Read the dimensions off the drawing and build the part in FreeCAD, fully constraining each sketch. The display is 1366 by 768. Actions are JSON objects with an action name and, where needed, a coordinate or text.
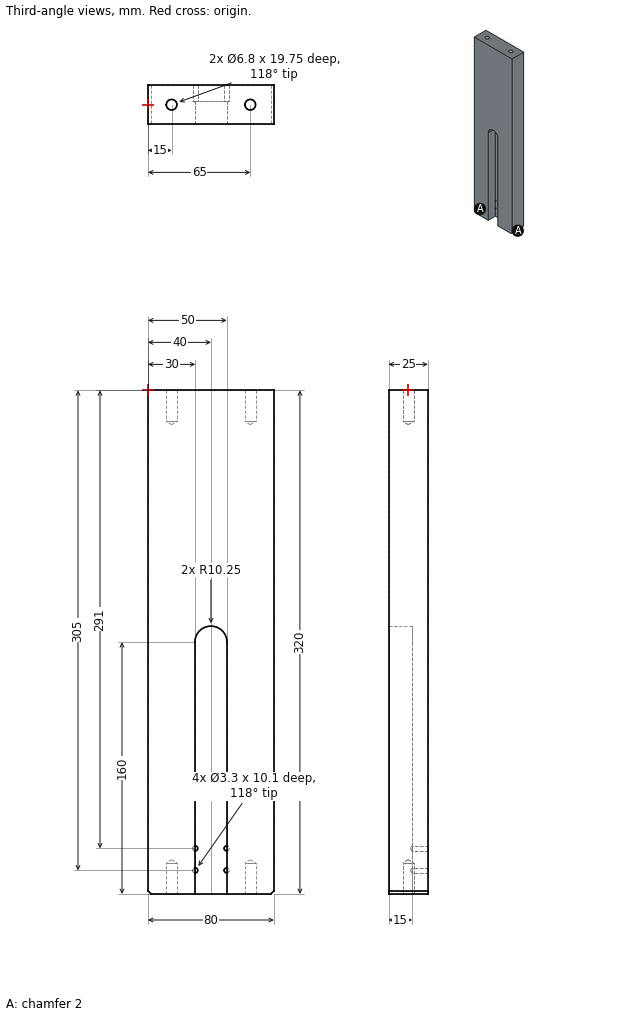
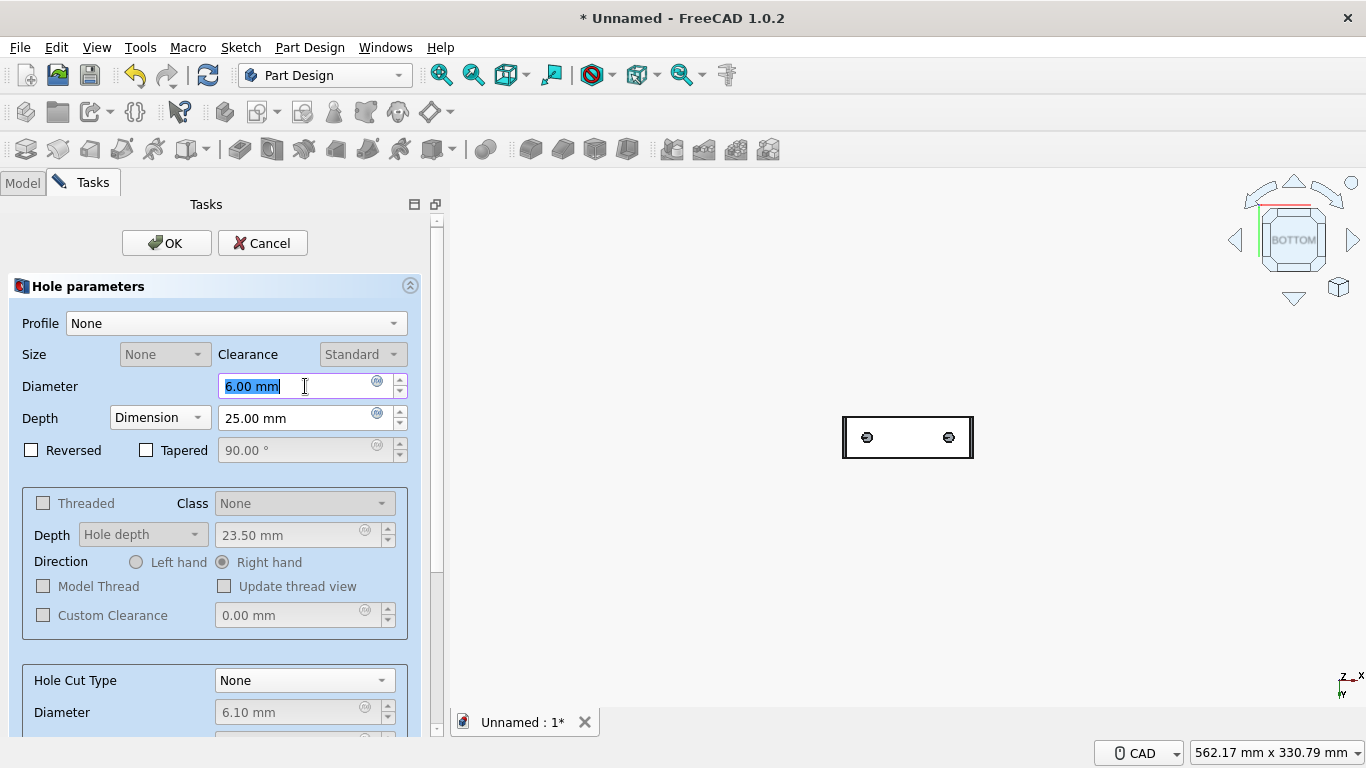
{"action": "type", "text": "6.8"}
{"action": "key", "text": "Tab"}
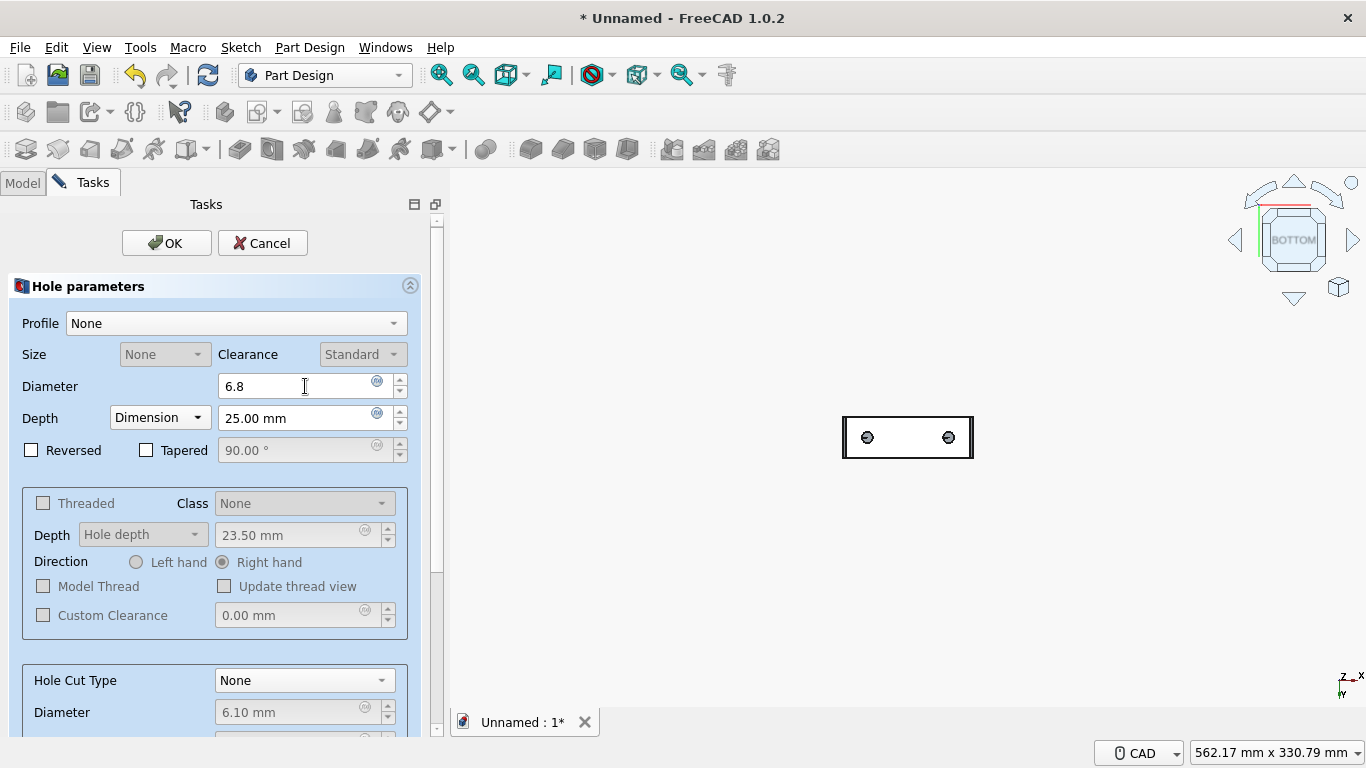
{"action": "triple_click", "coordinate": [305, 418]}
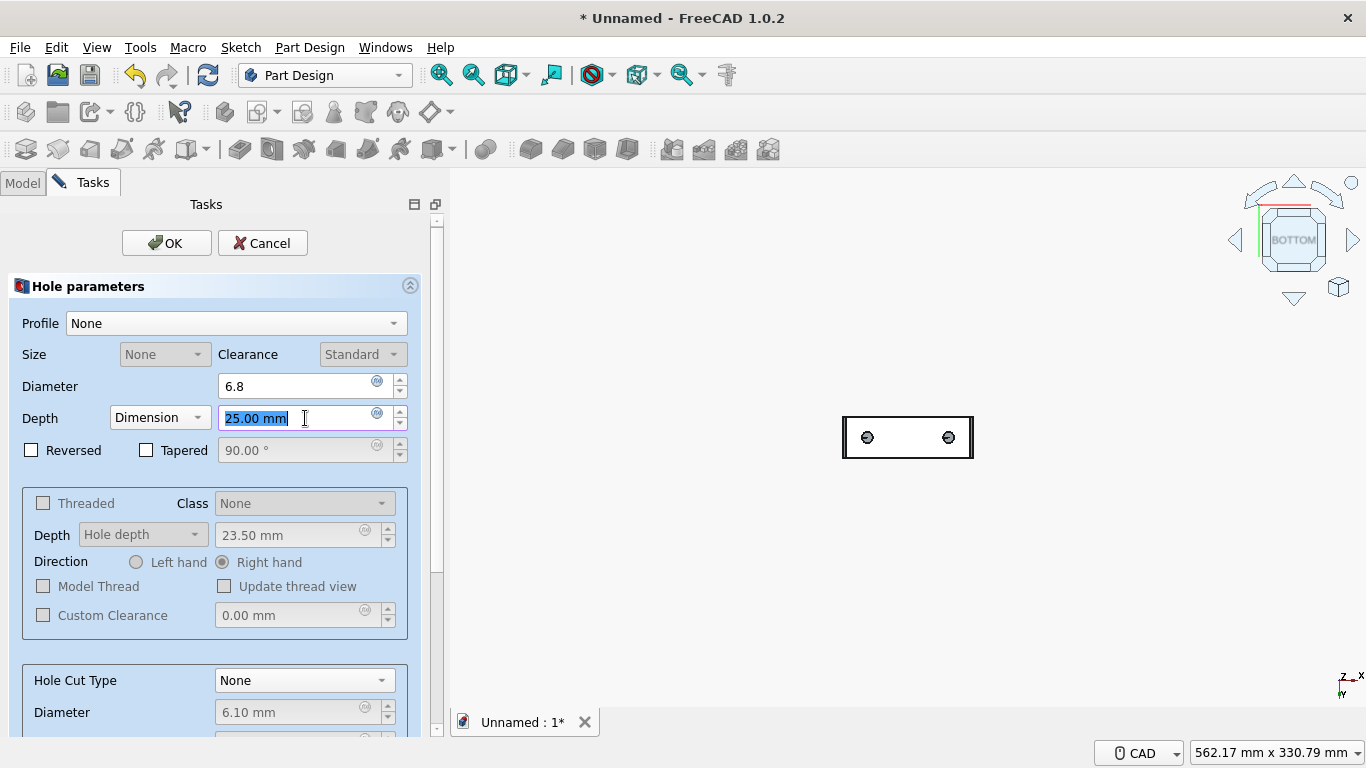
{"action": "type", "text": "19.75"}
{"action": "key", "text": "Tab"}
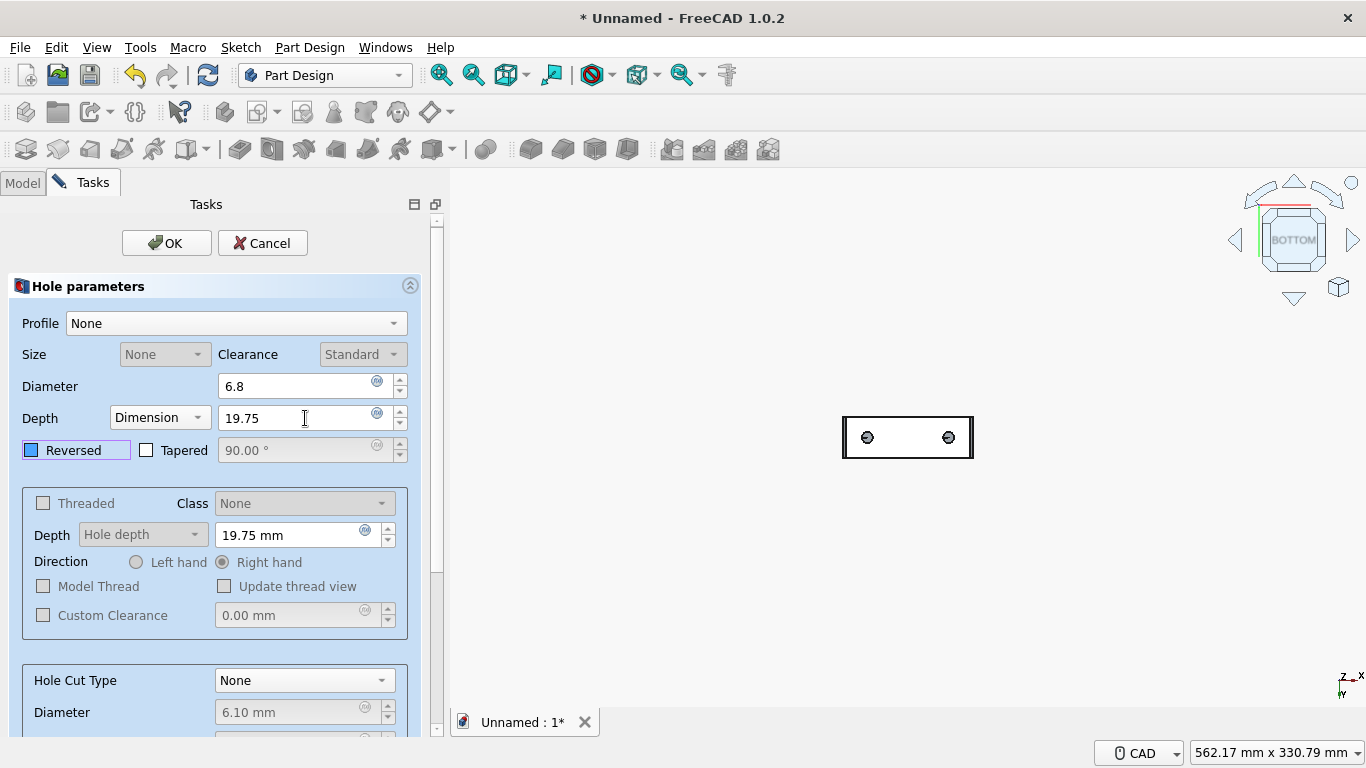
{"action": "left_click", "coordinate": [167, 243]}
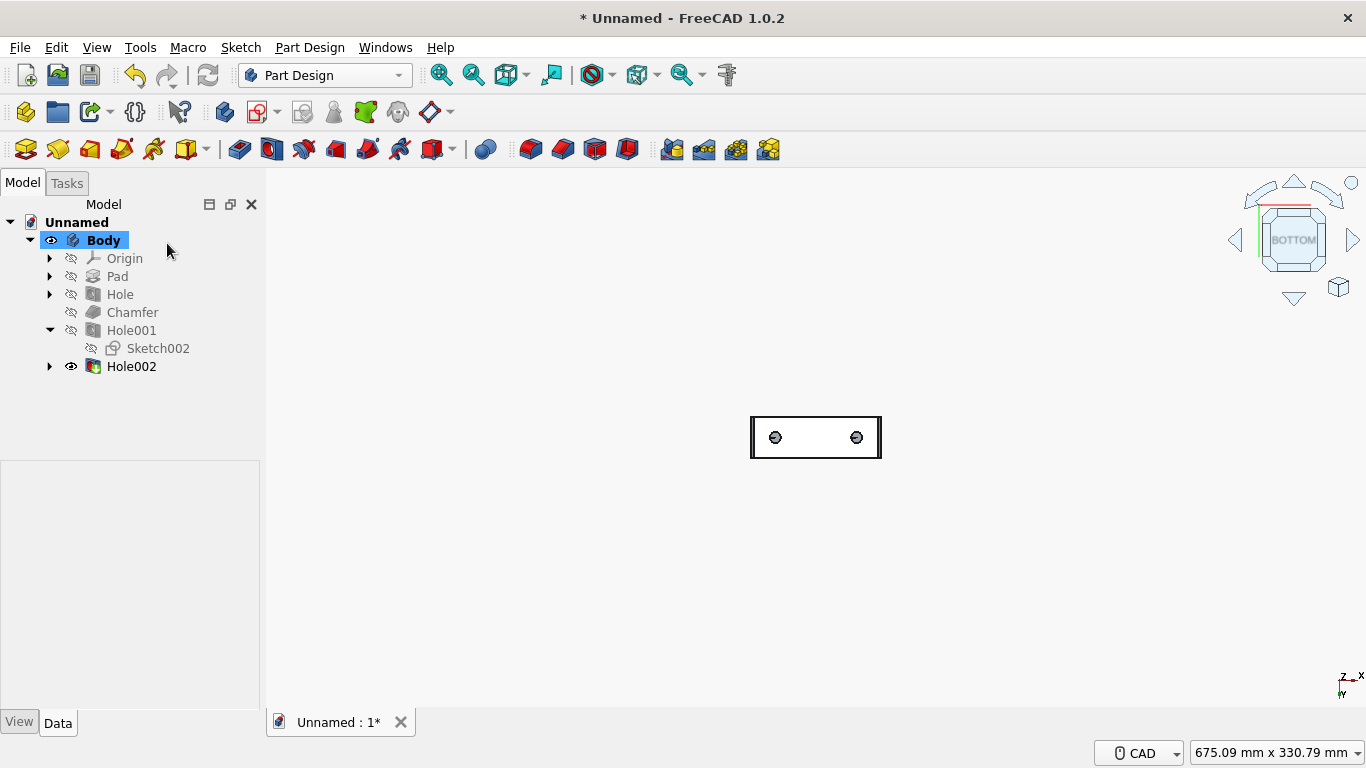
{"action": "left_click", "coordinate": [442, 76]}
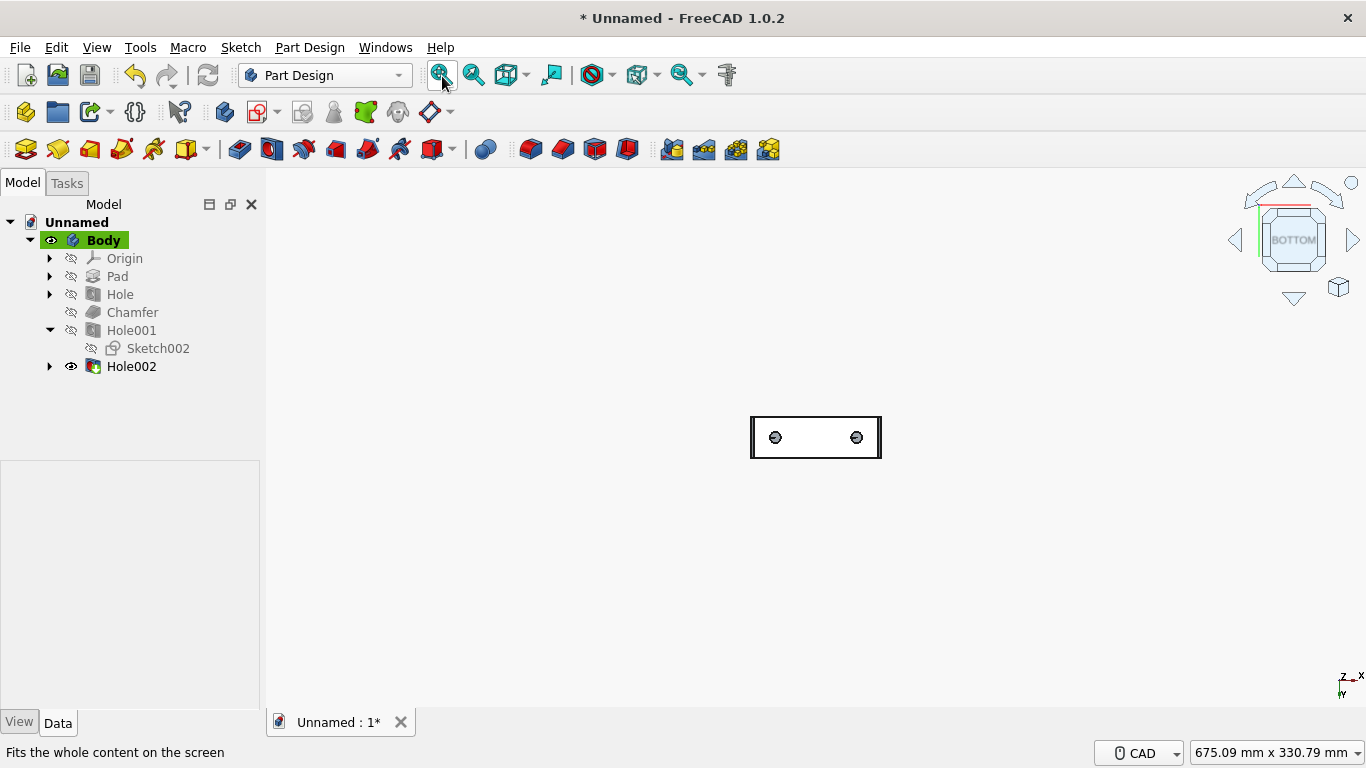
{"action": "key", "text": "0"}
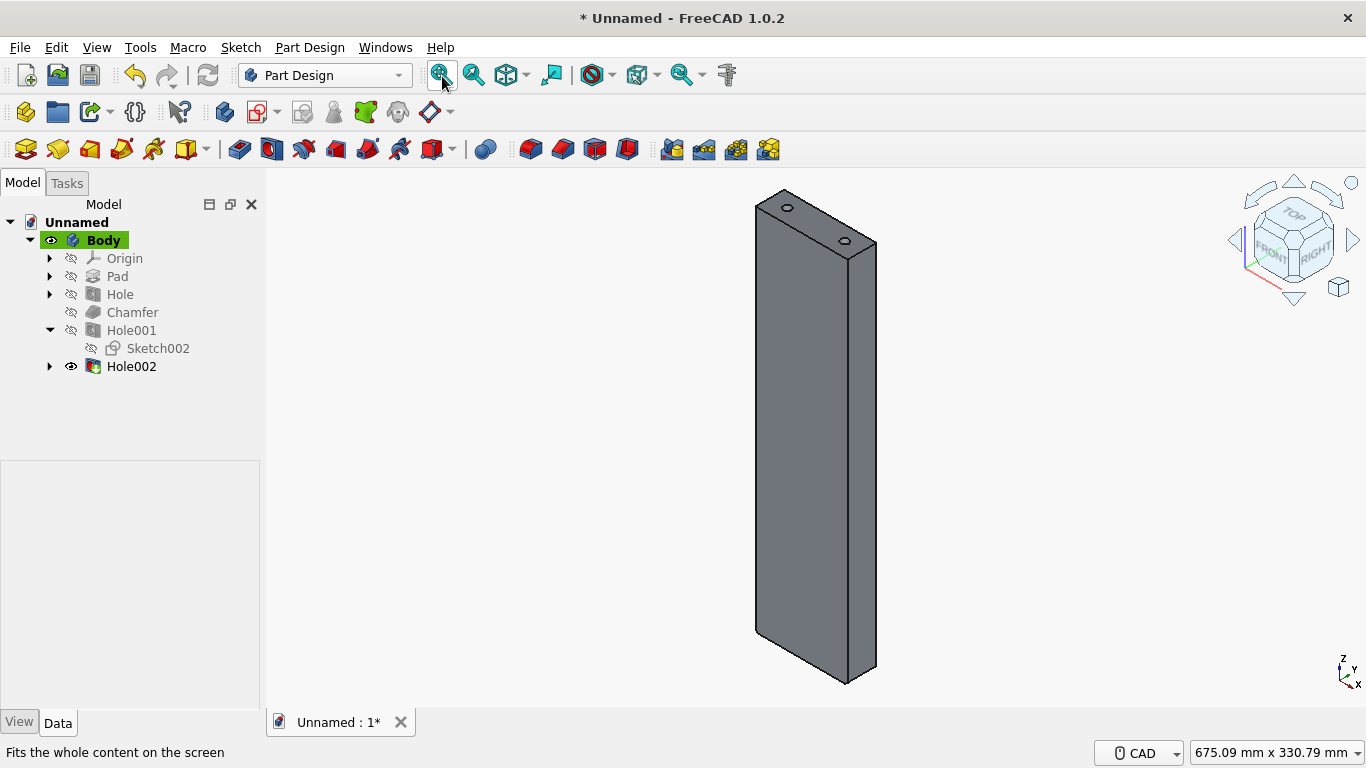
{"action": "left_click", "coordinate": [802, 323]}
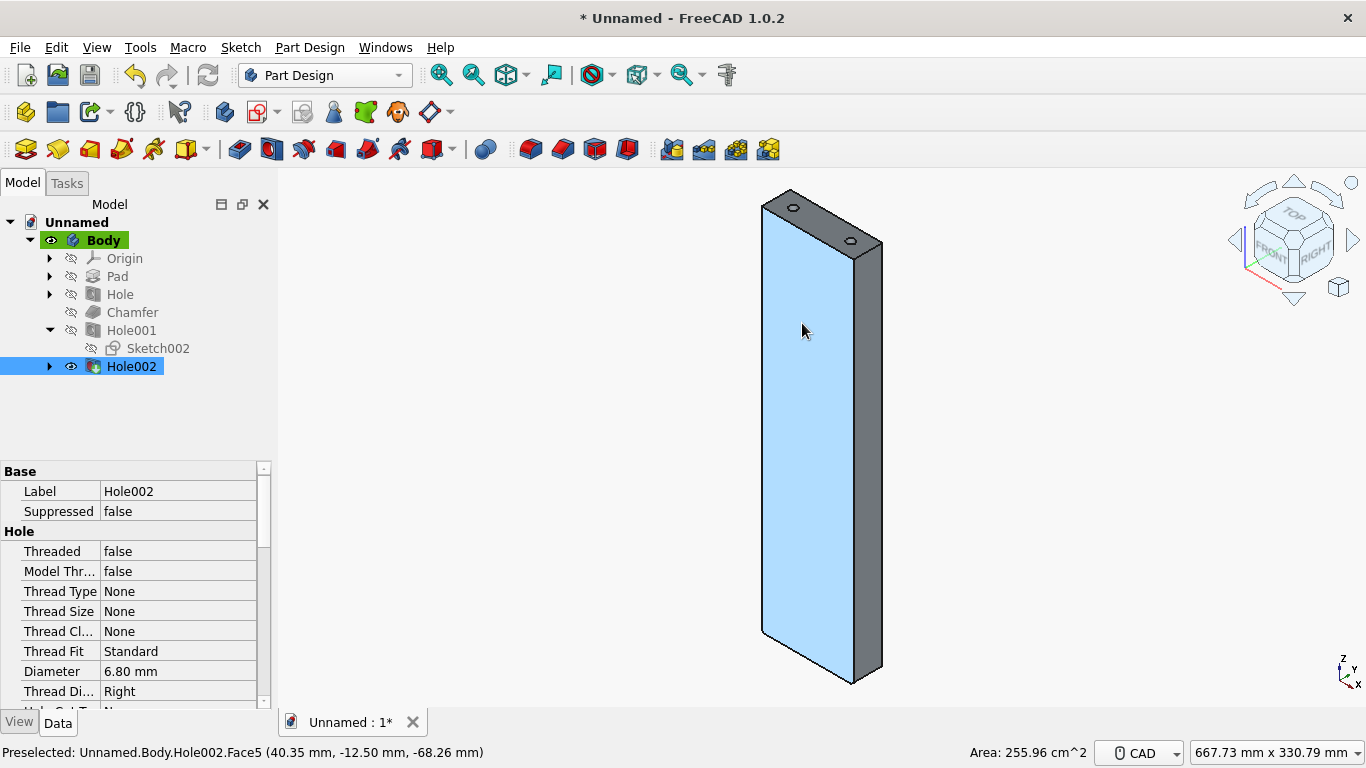
{"action": "left_click", "coordinate": [258, 112]}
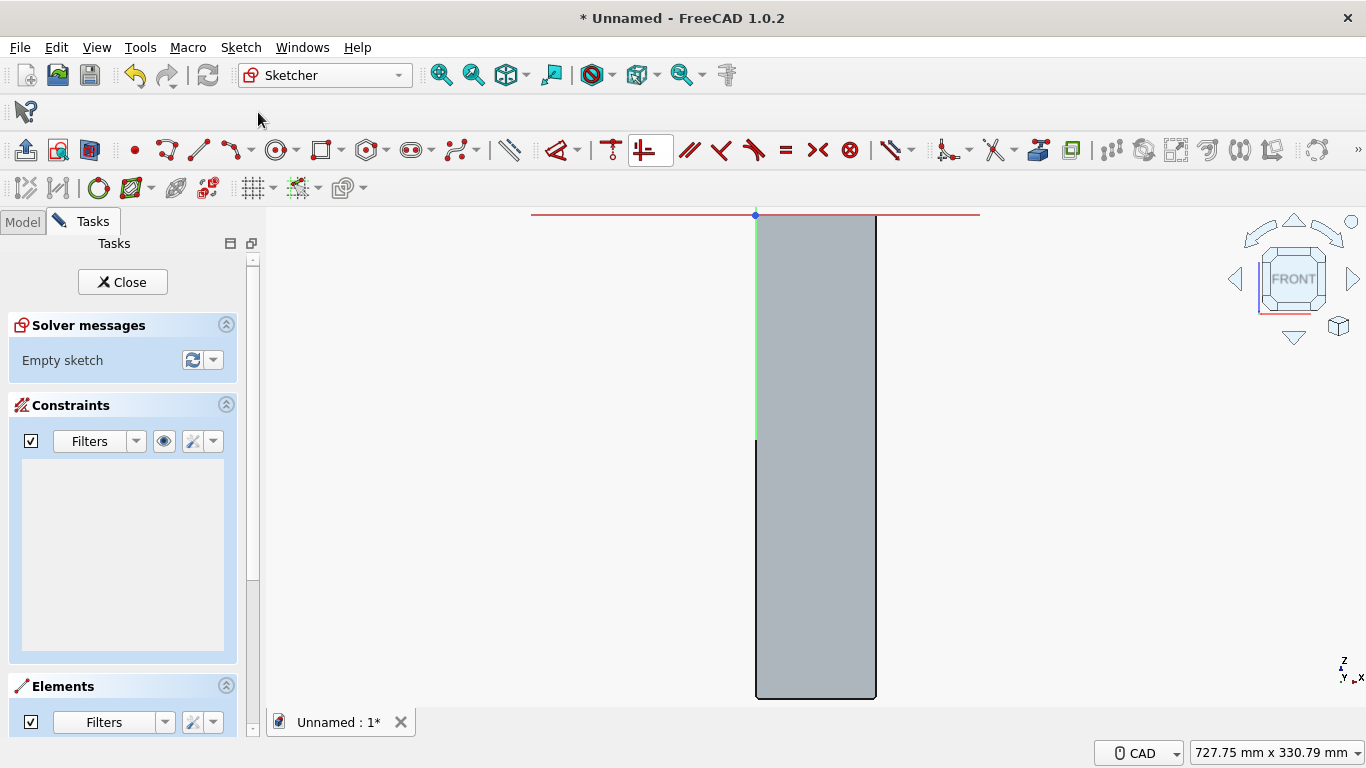
{"action": "scroll", "coordinate": [654, 441], "scroll_direction": "down", "scroll_amount": 2}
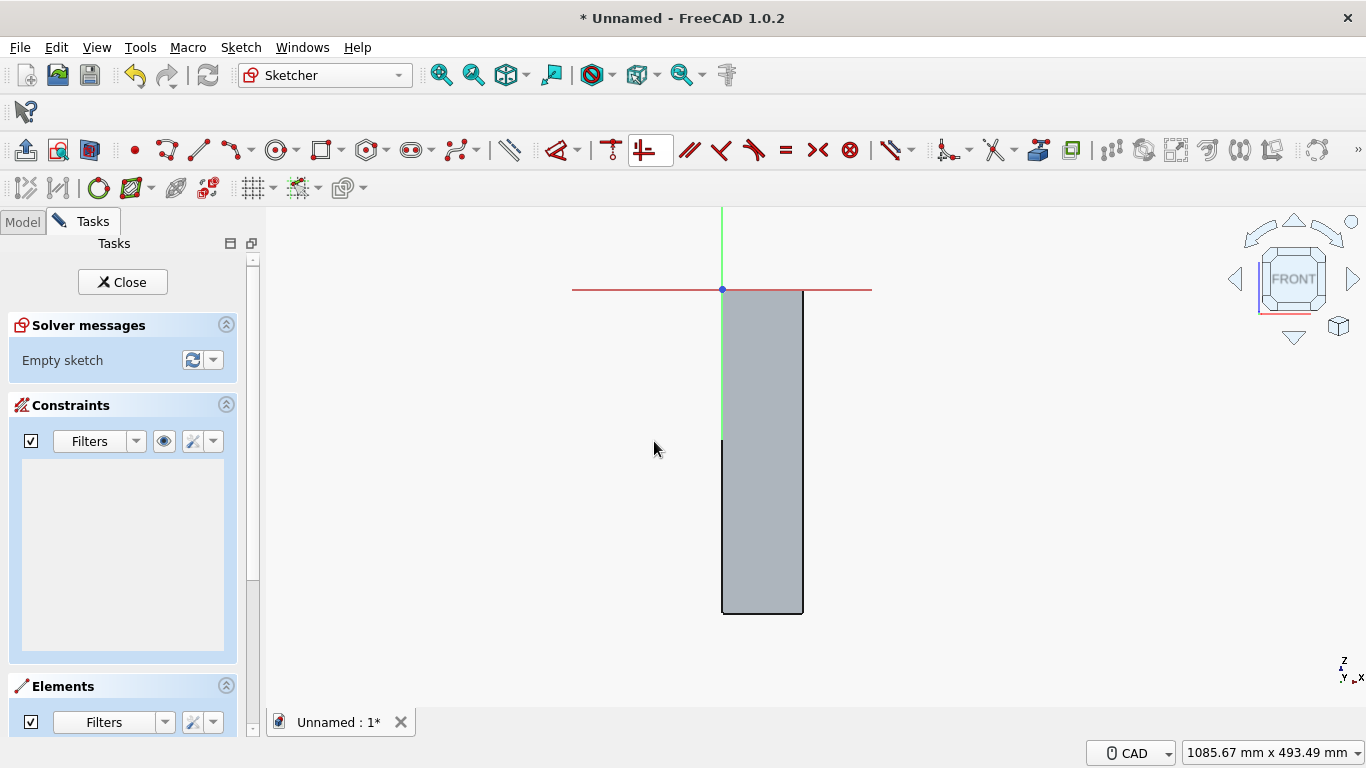
{"action": "left_click", "coordinate": [412, 150]}